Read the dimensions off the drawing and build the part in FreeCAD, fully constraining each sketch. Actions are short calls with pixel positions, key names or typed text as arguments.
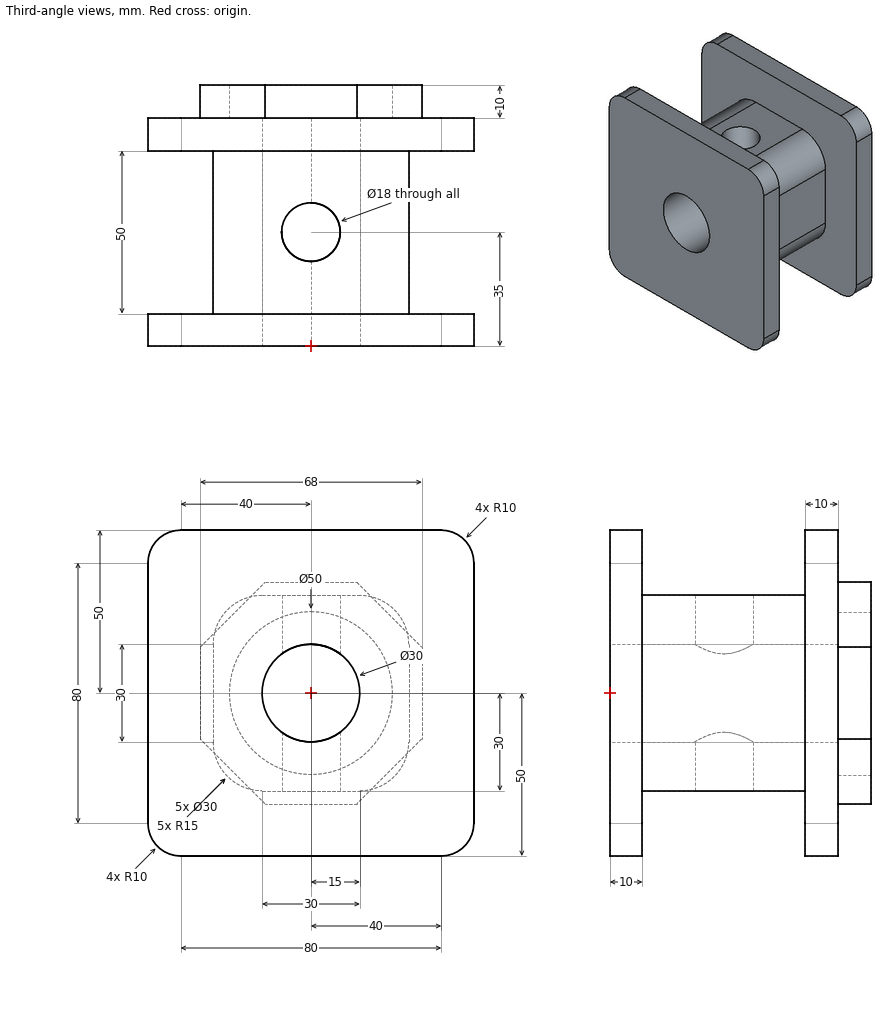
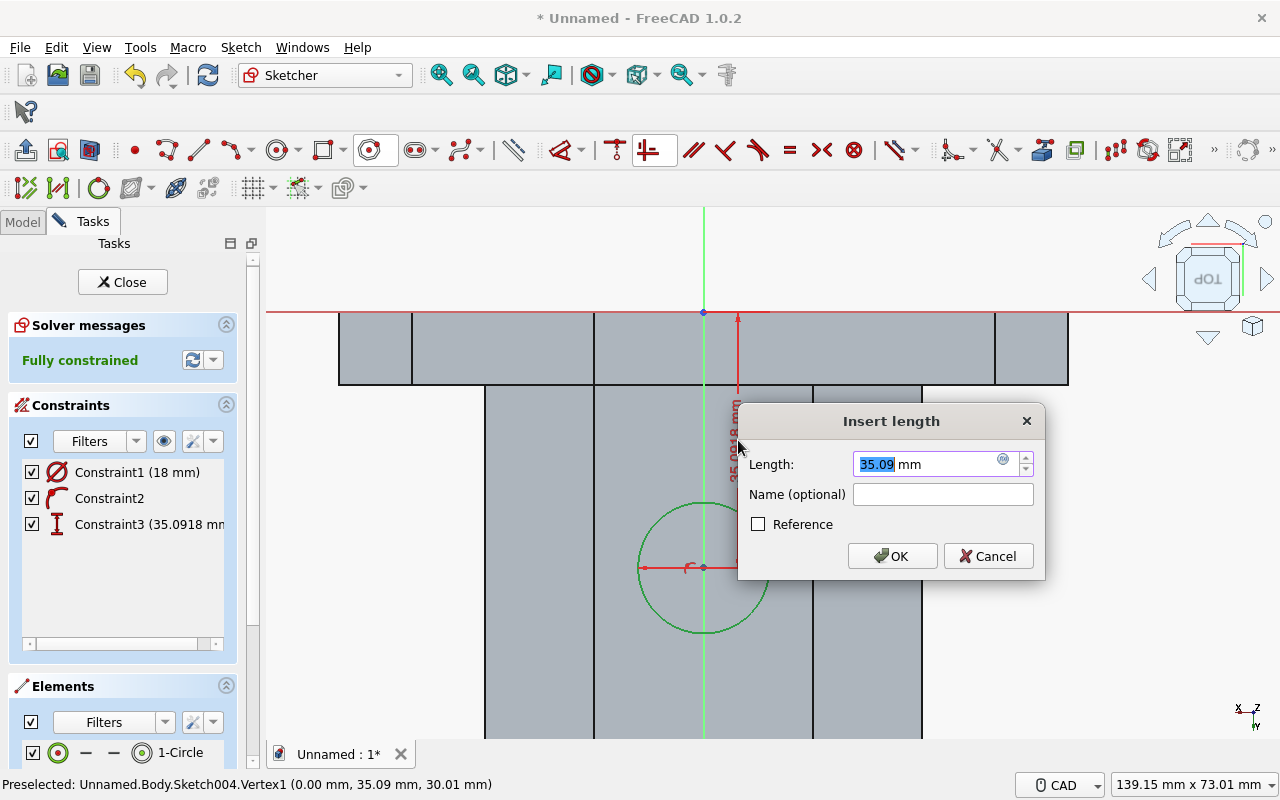
text(35)
key(Return)
key(Escape)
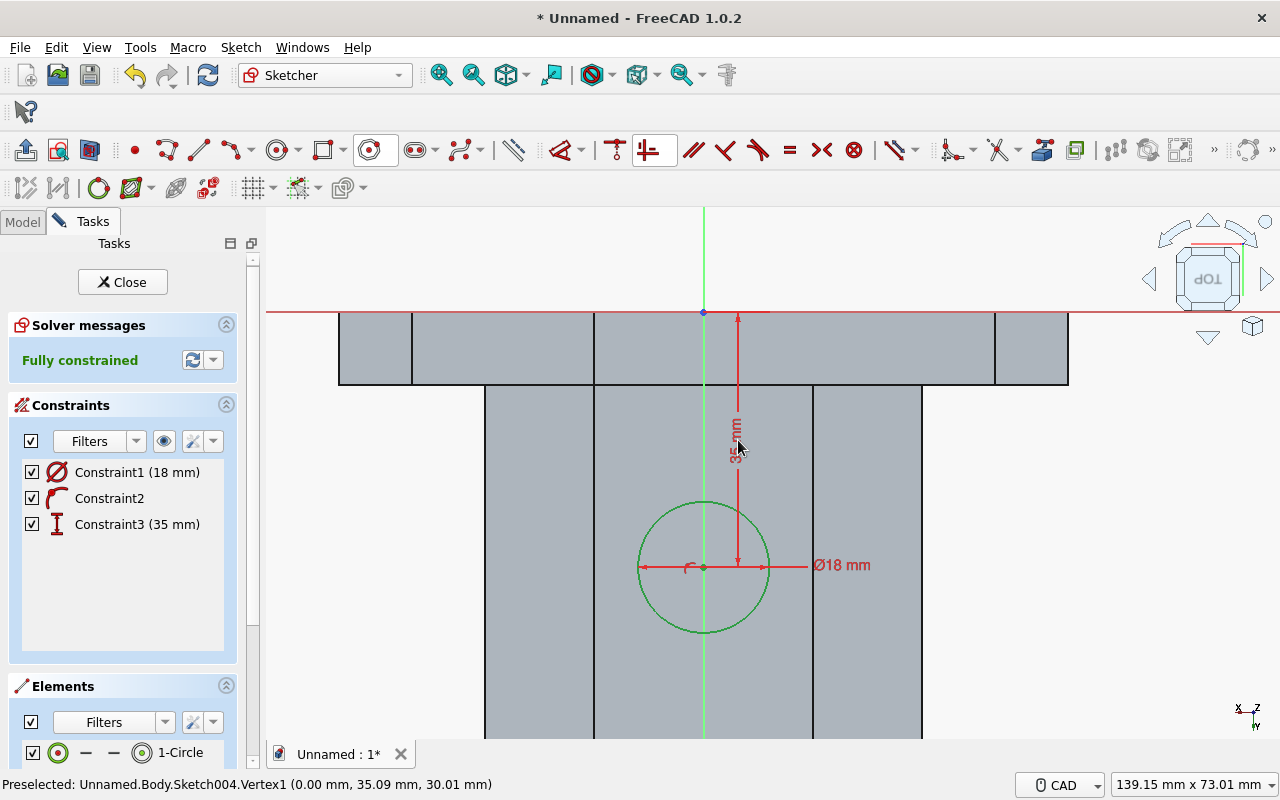
click(123, 282)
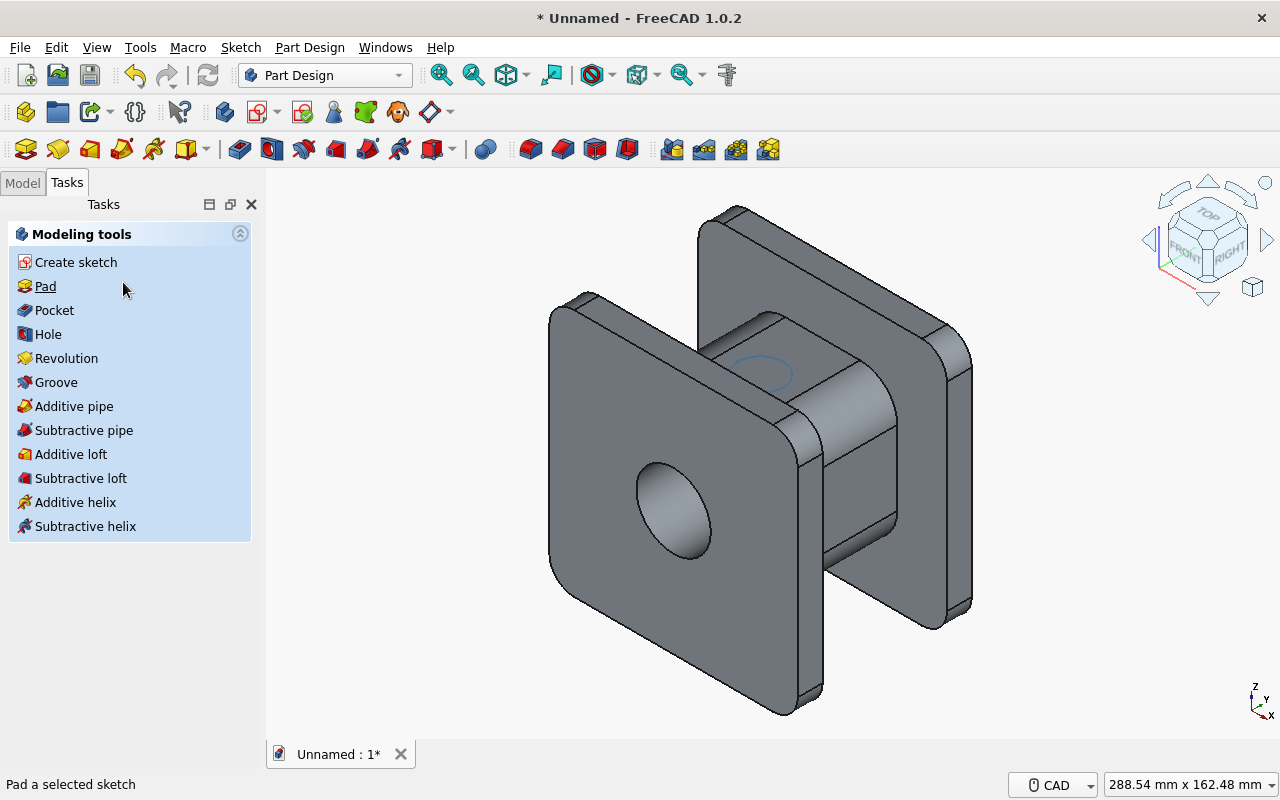
click(272, 150)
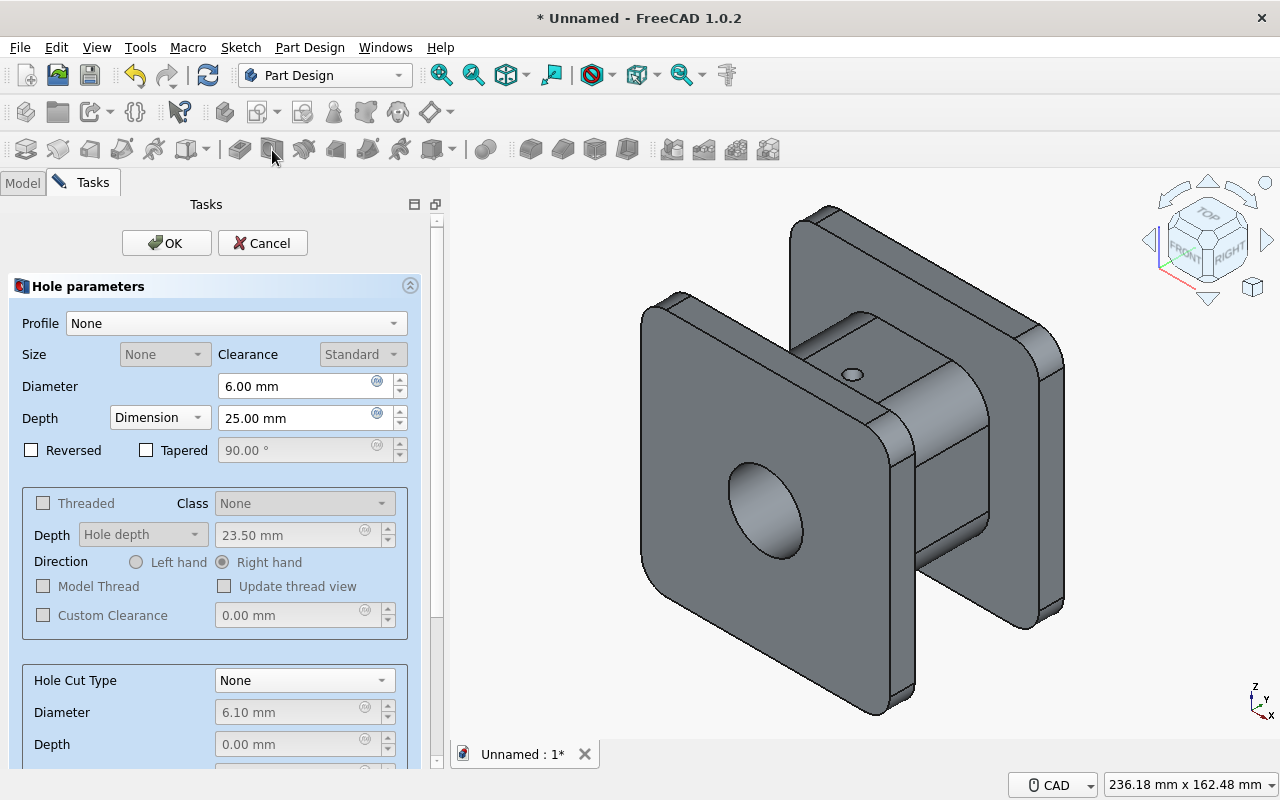
triple_click(305, 386)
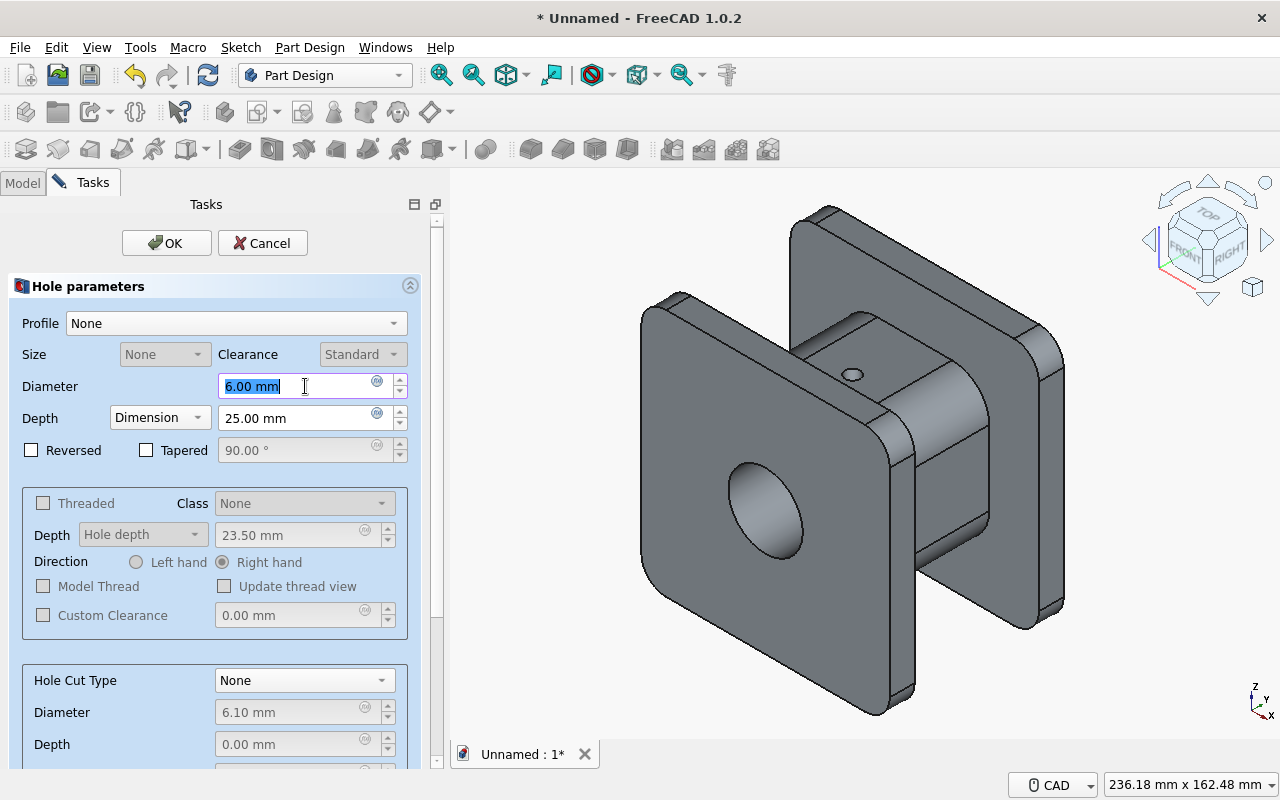
text(18)
key(Tab)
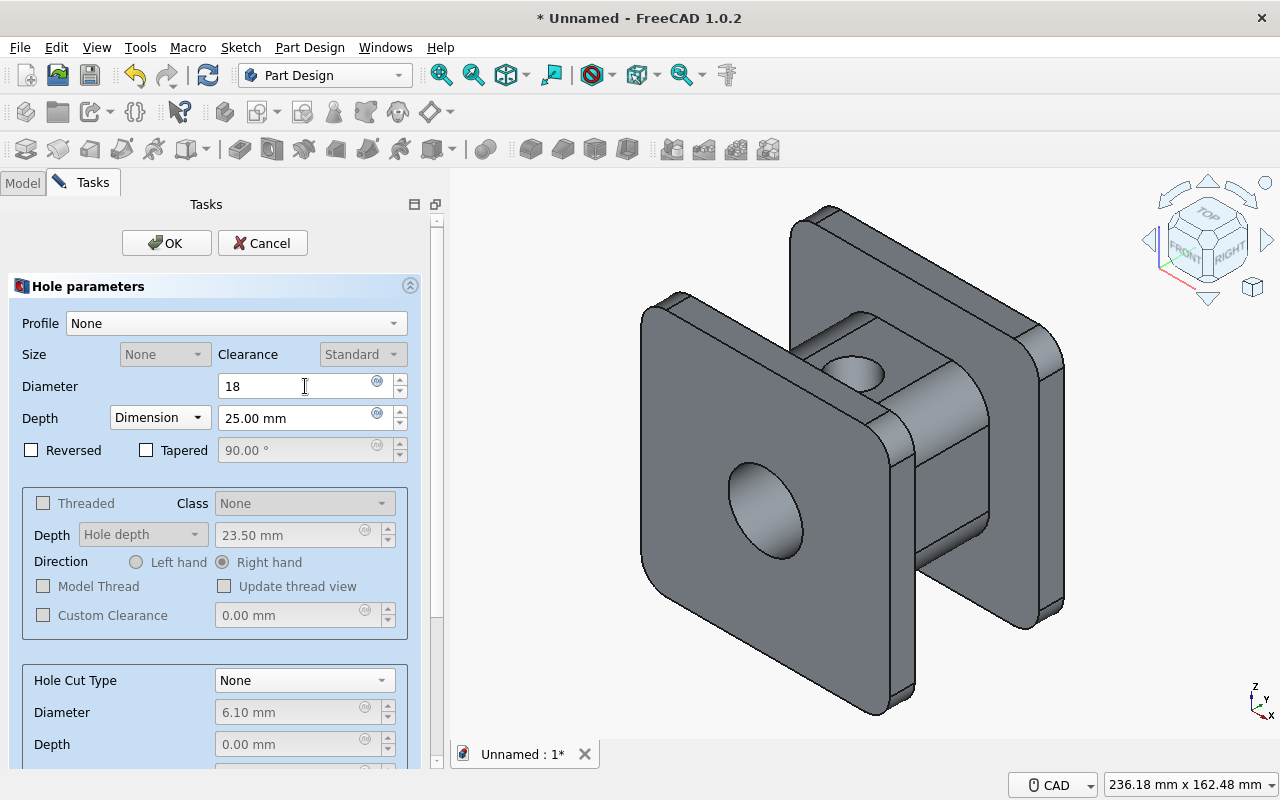
click(161, 418)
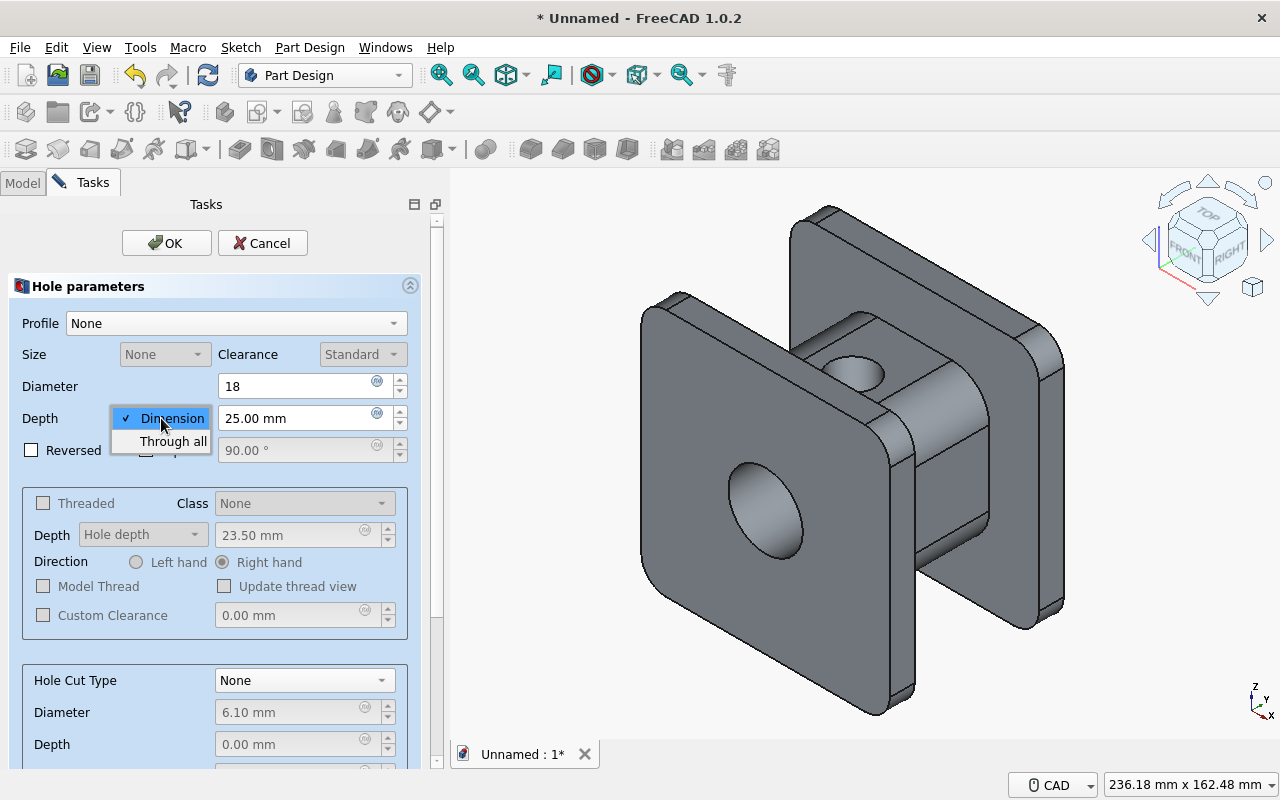
click(160, 442)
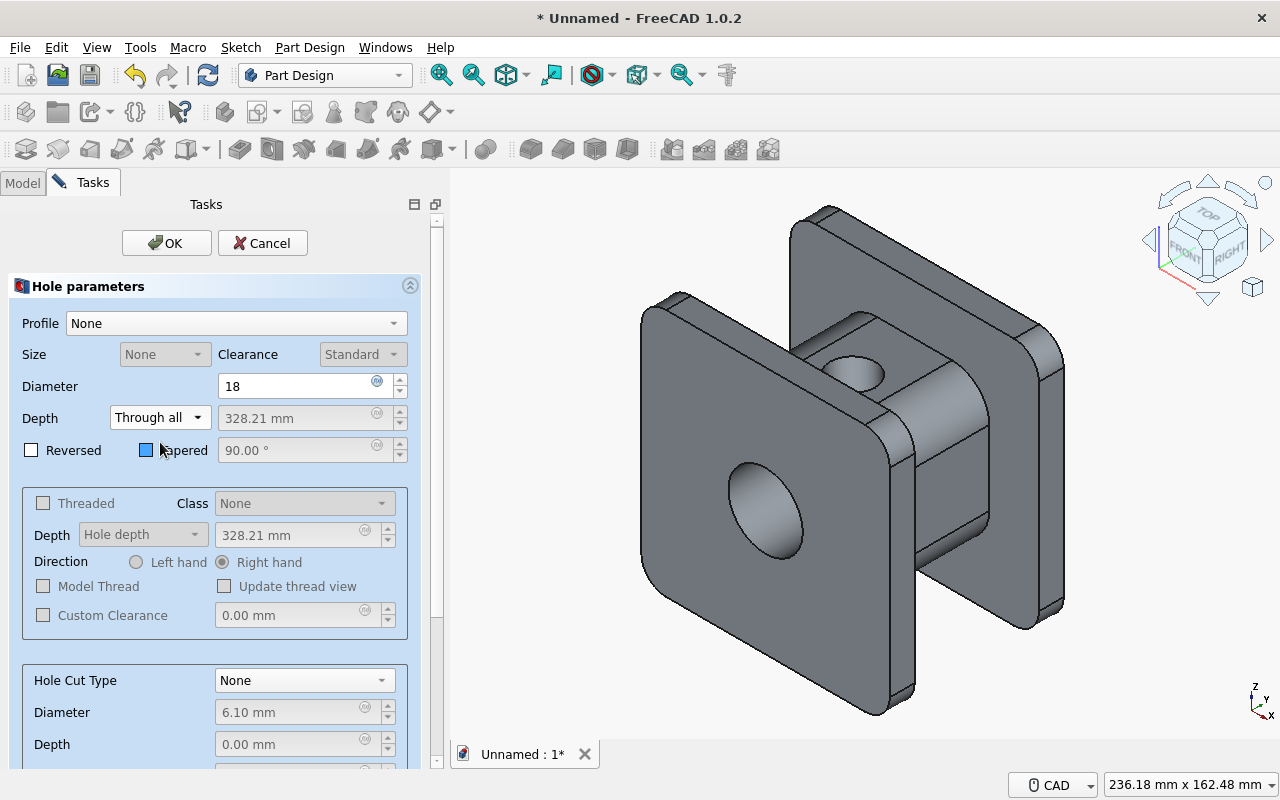
click(167, 243)